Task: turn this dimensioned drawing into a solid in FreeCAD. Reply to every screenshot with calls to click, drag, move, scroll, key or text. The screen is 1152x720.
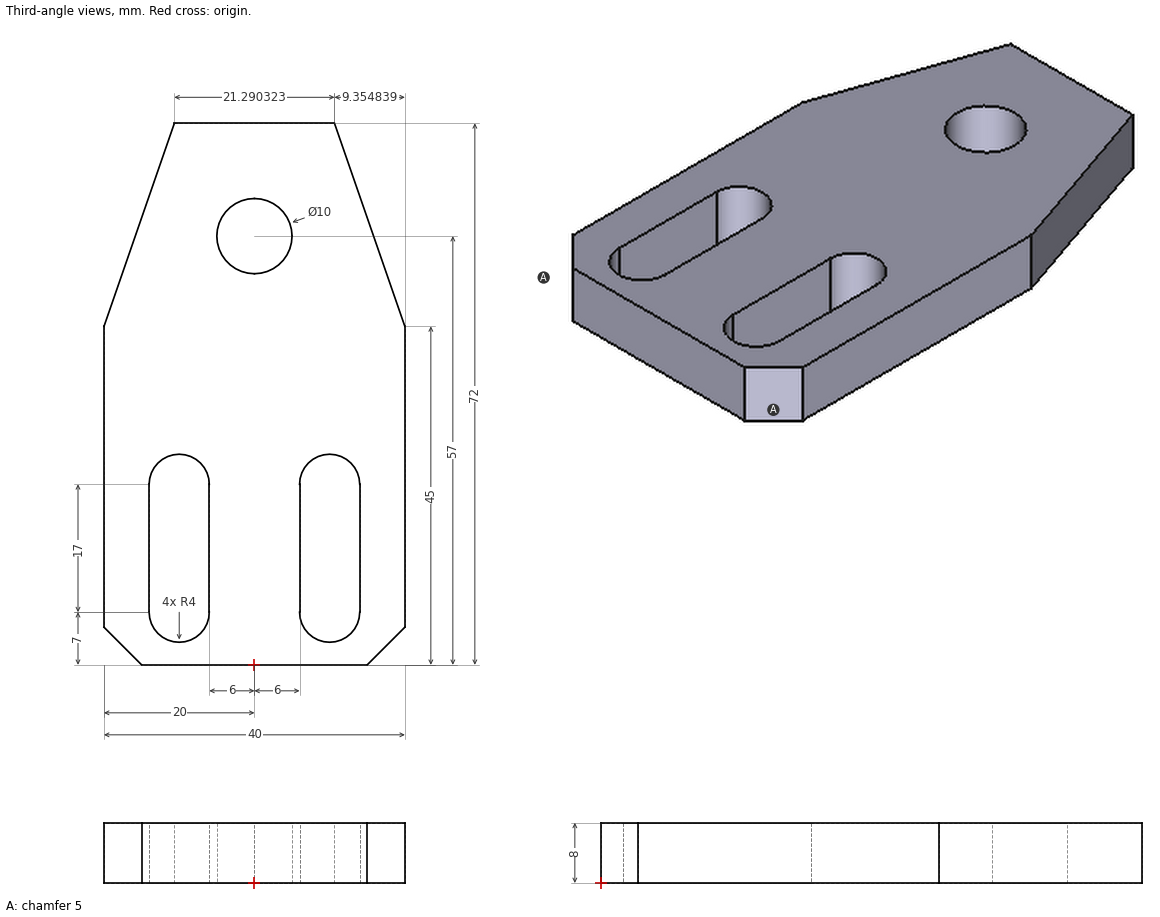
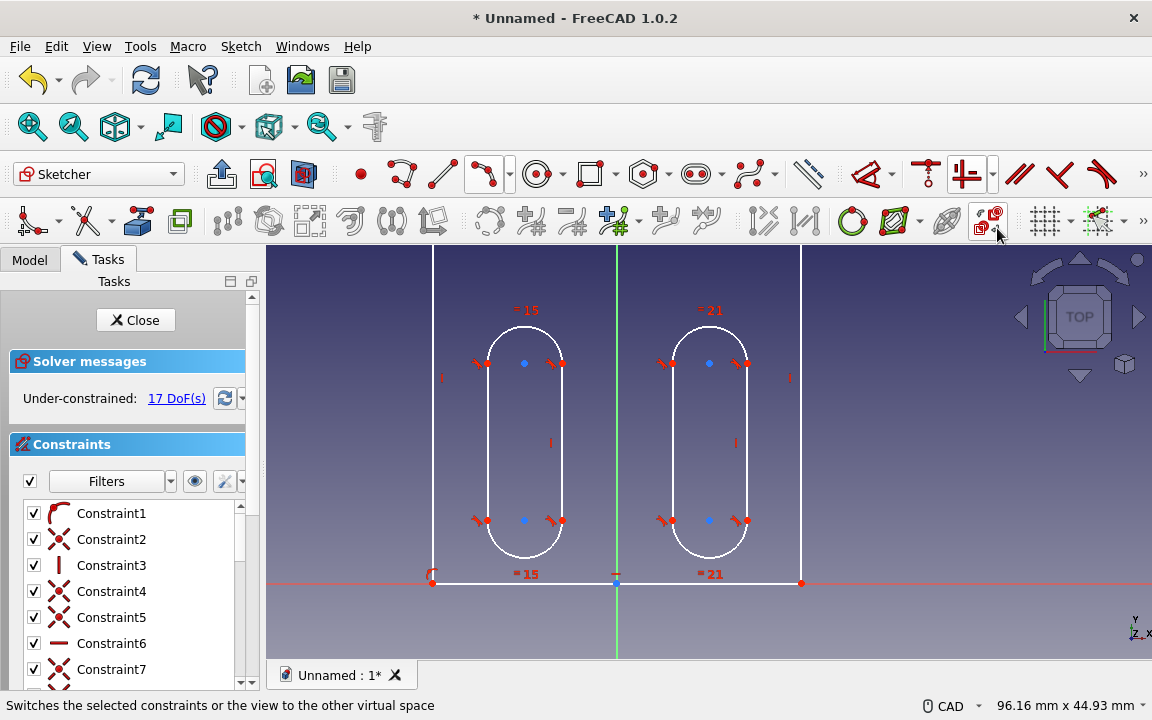
click(503, 551)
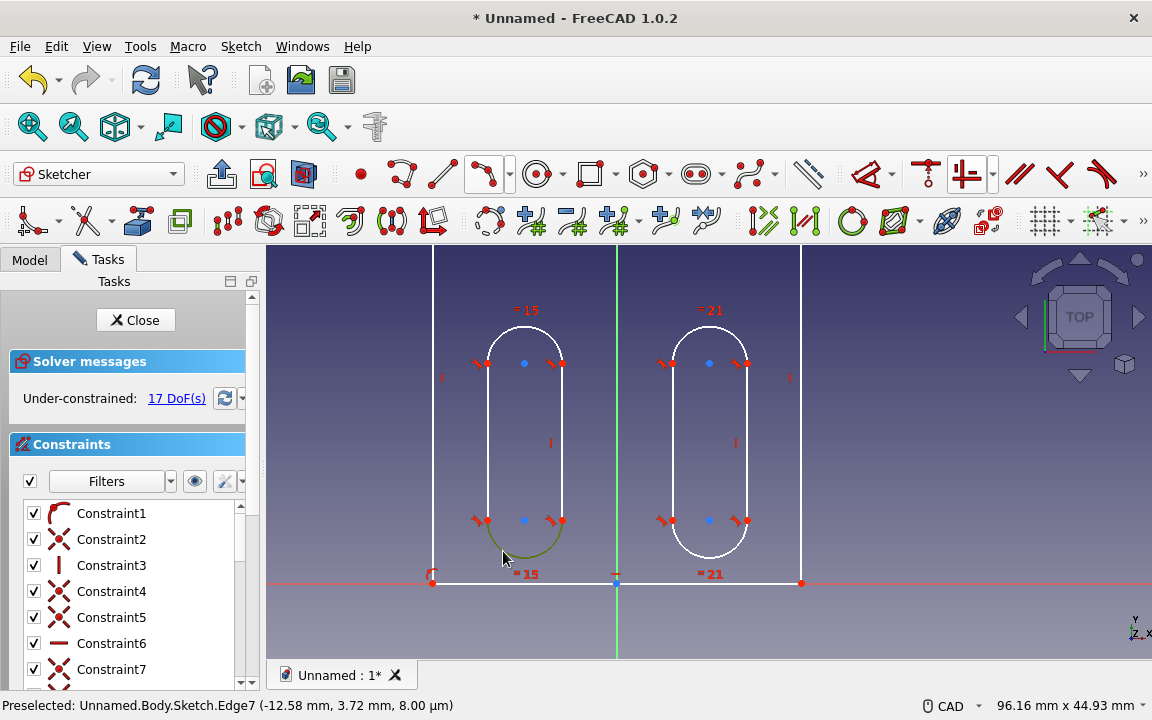
click(688, 551)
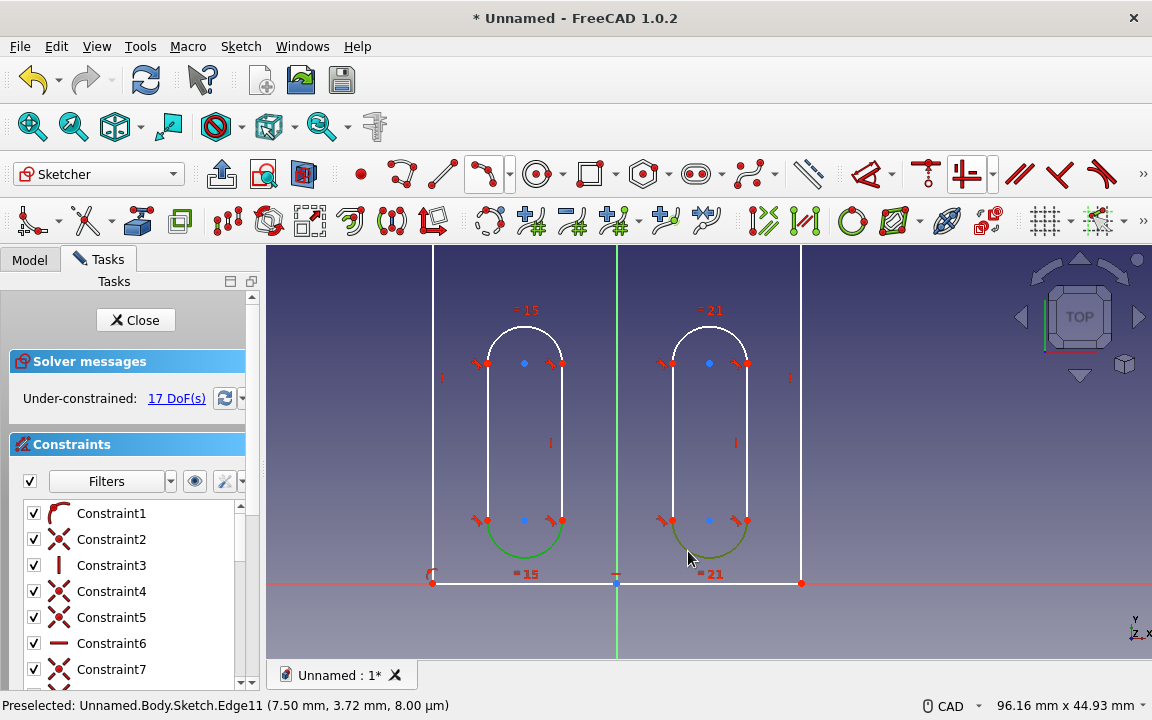
key(e)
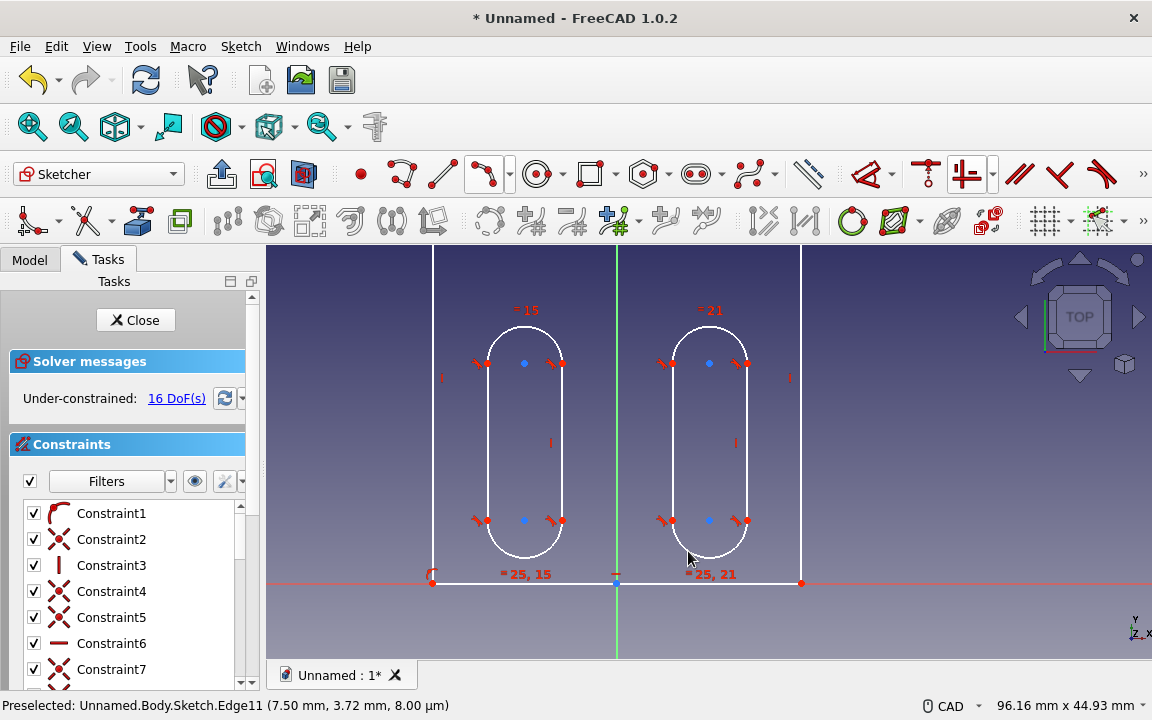
click(866, 174)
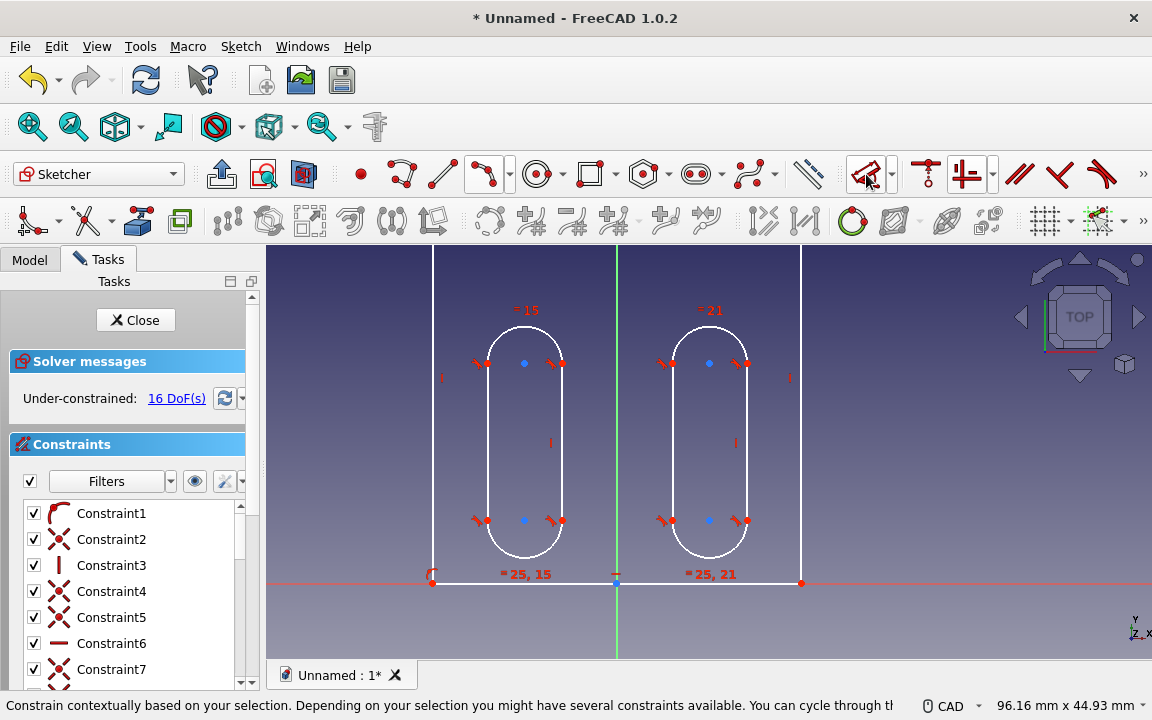
click(503, 551)
click(462, 551)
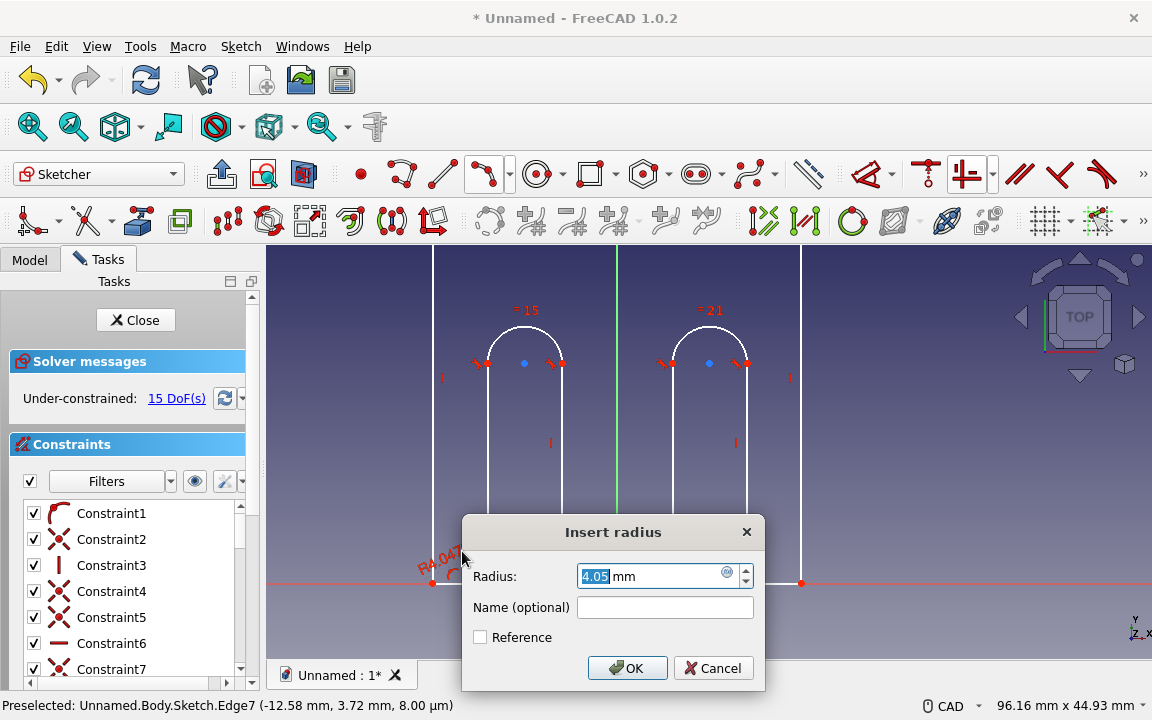
text(4)
key(Return)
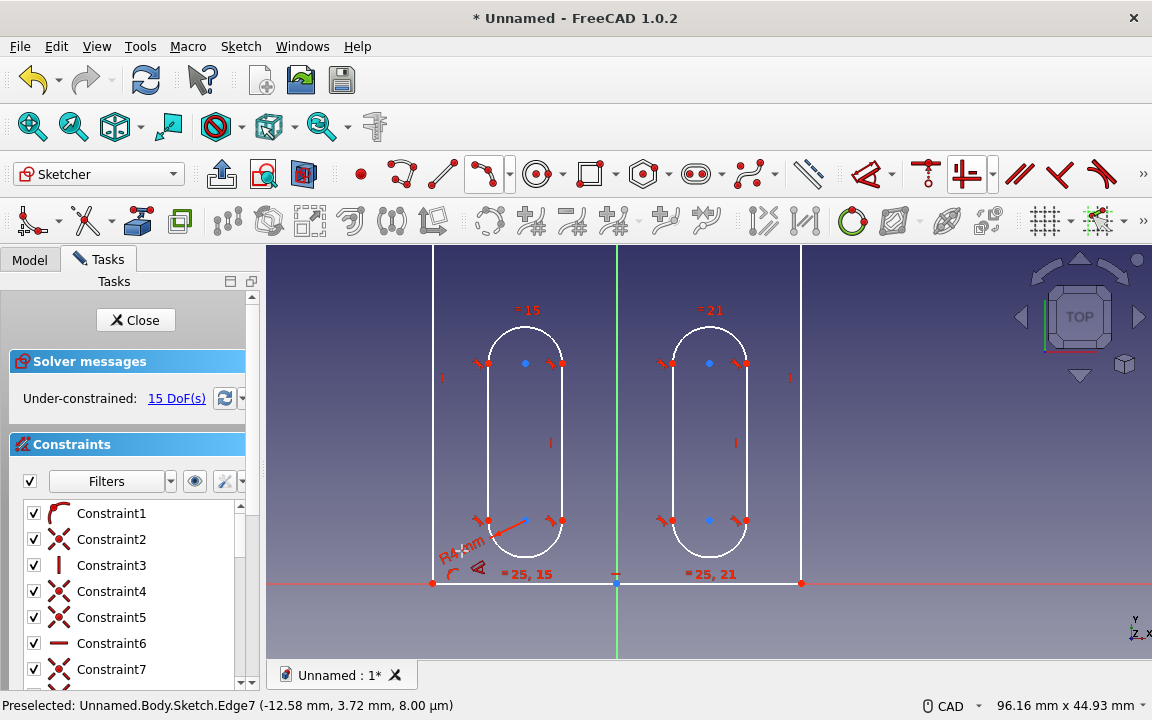
scroll(654, 568, down, 5)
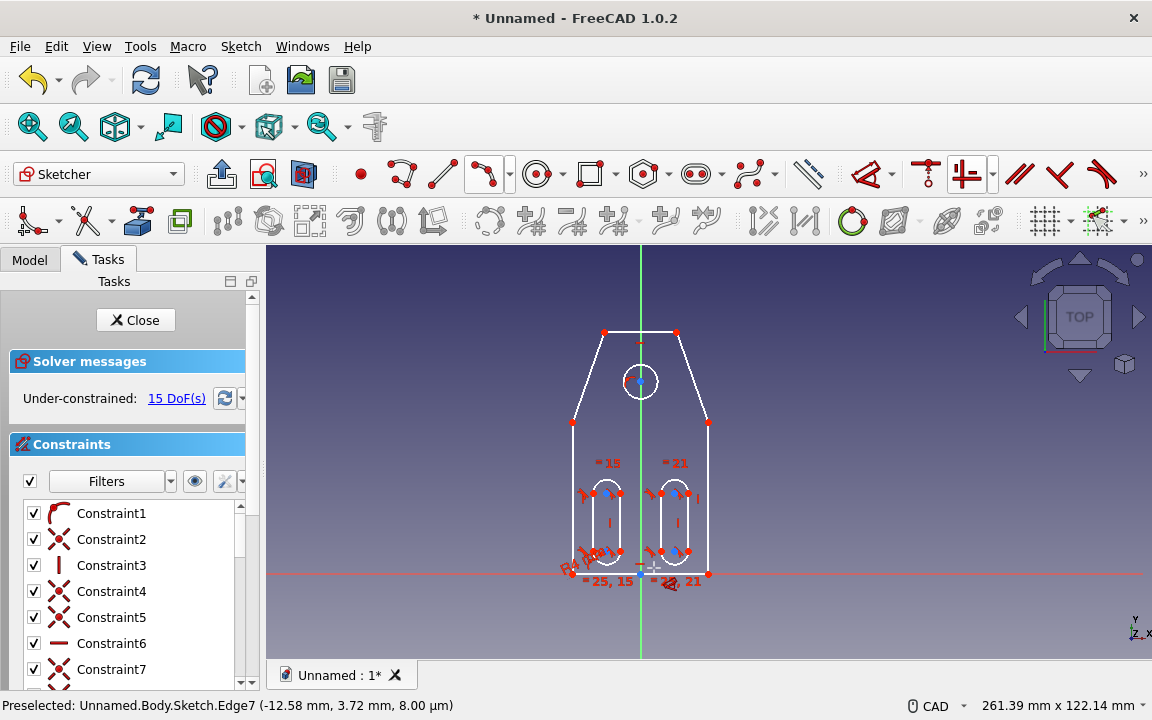
click(653, 370)
click(675, 417)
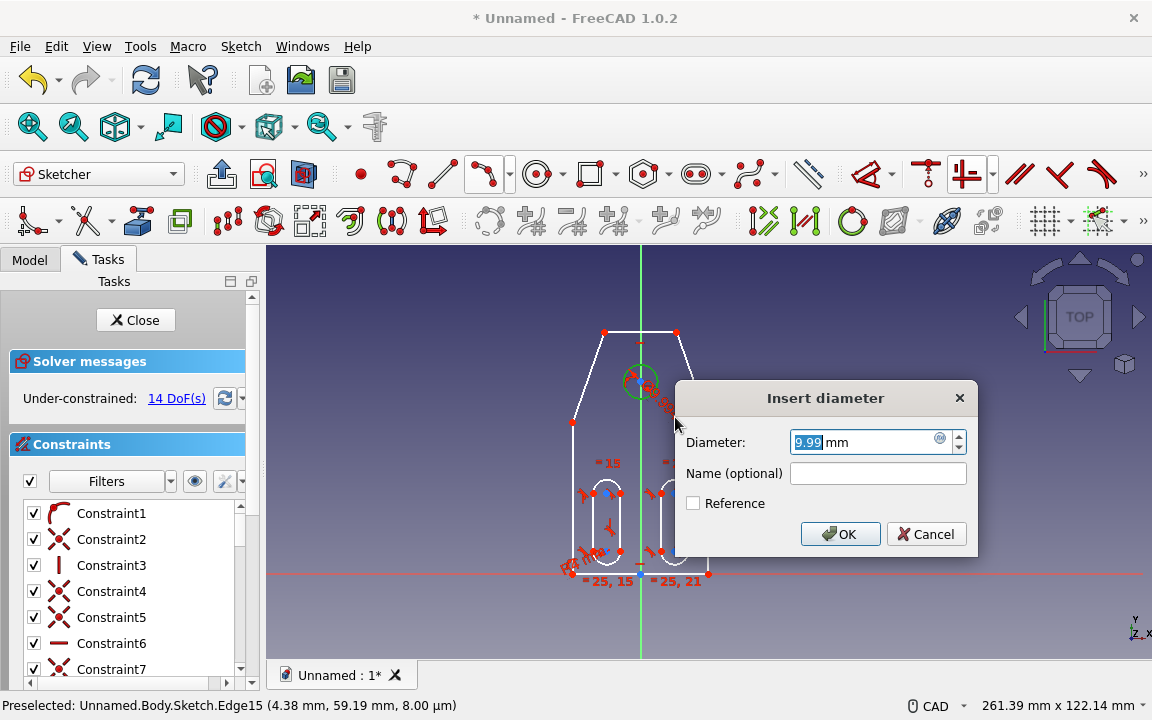
text(10)
key(Return)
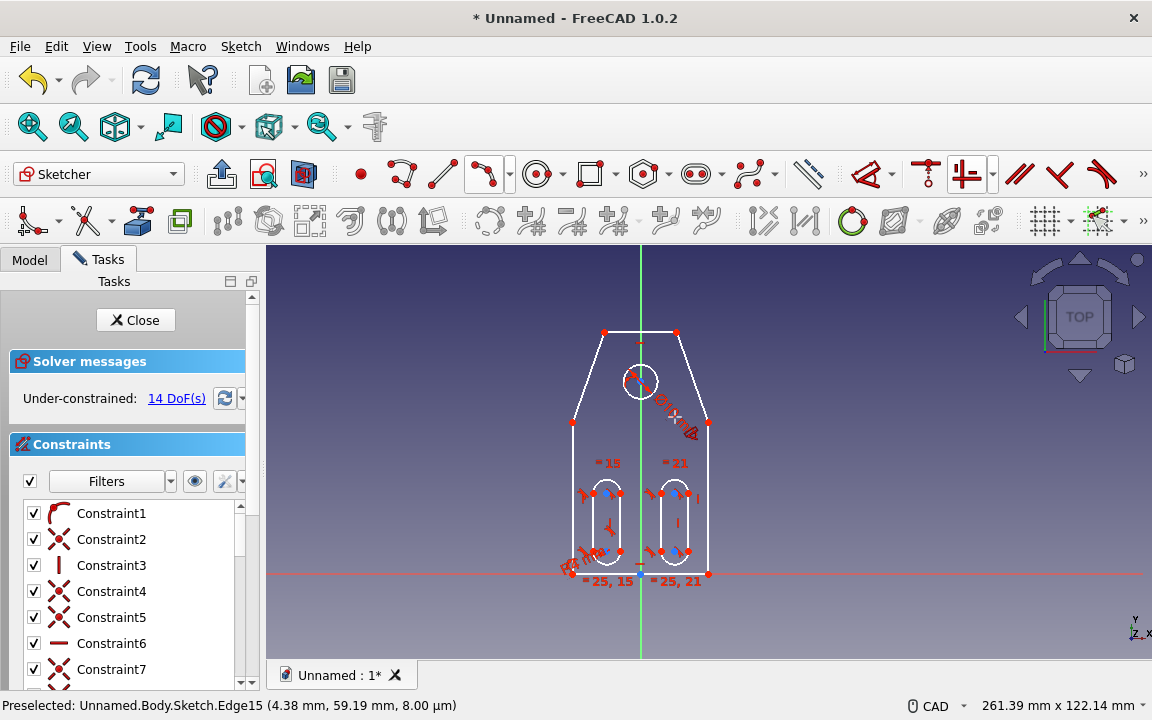
scroll(614, 574, up, 2)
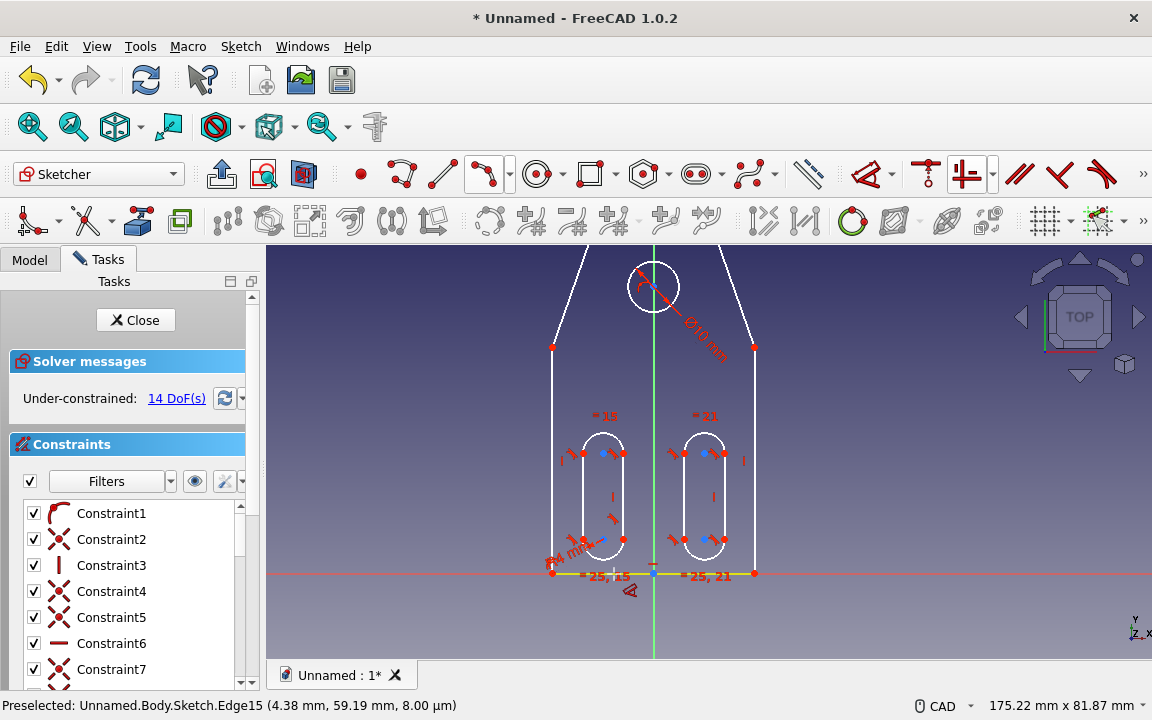
click(613, 574)
click(607, 608)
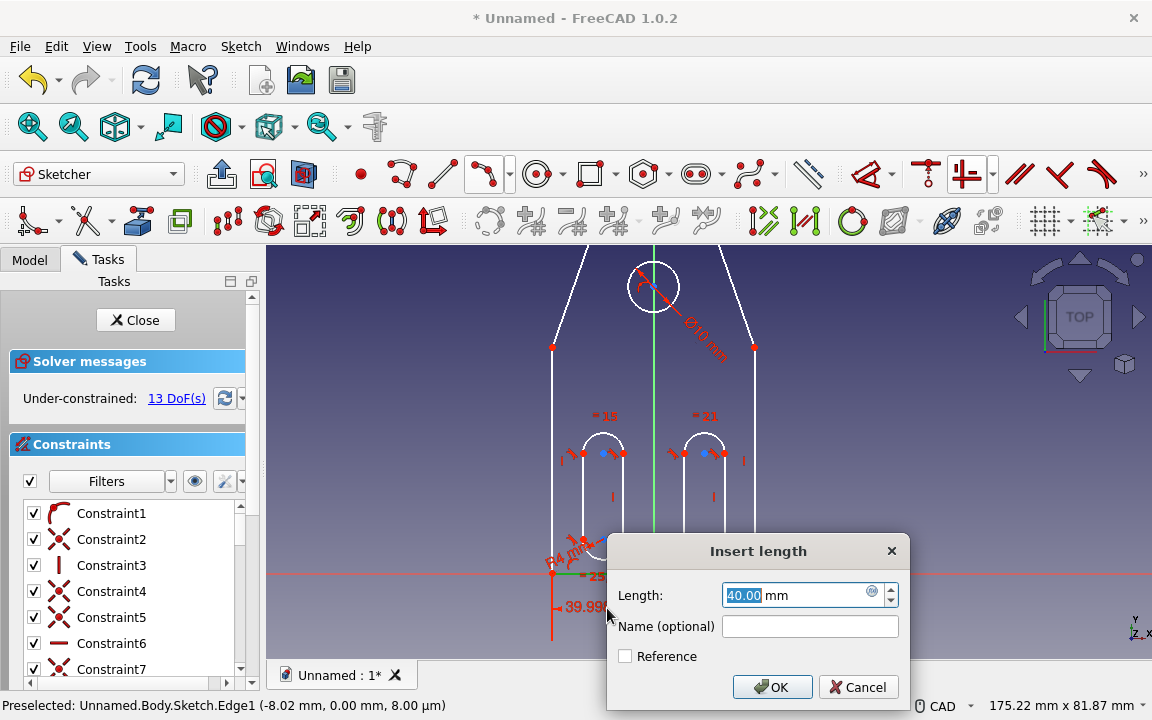
text(40)
key(Return)